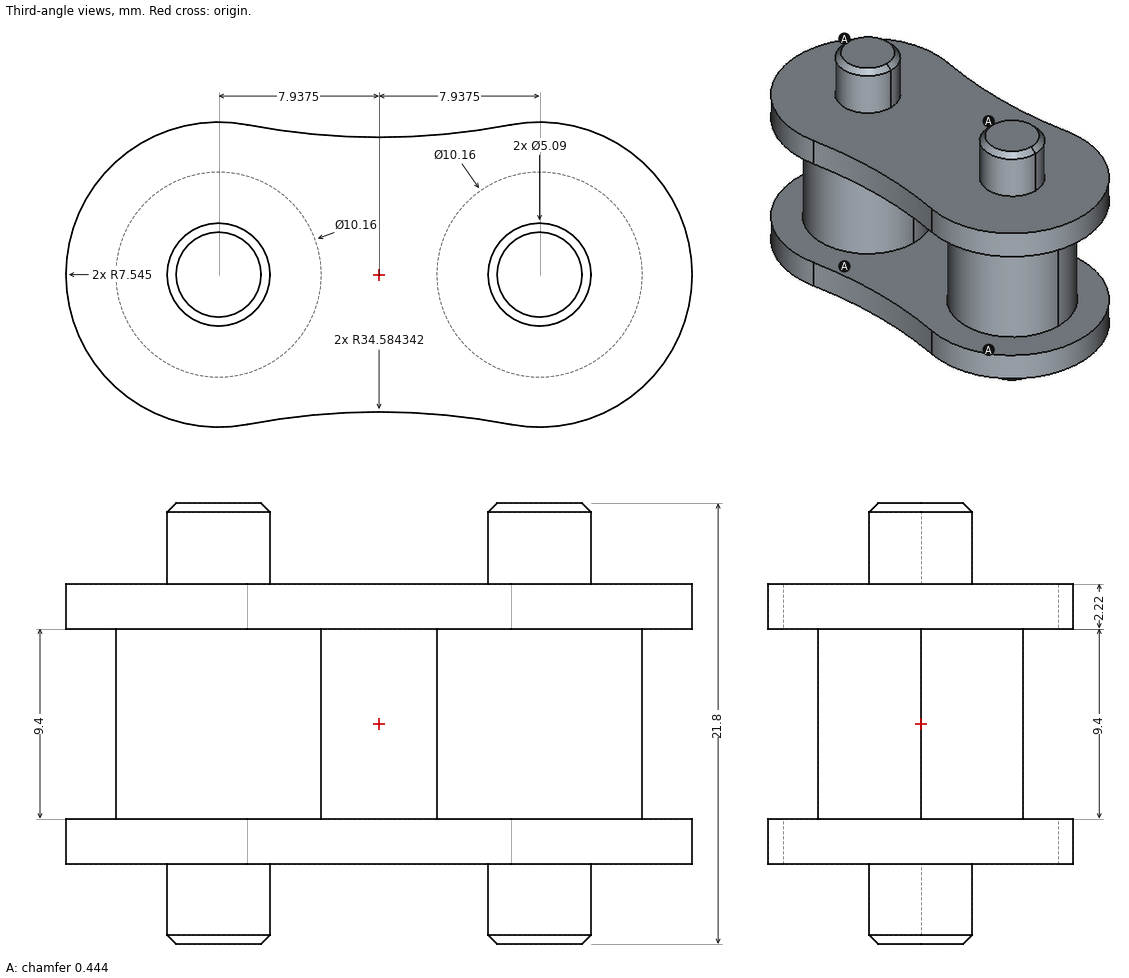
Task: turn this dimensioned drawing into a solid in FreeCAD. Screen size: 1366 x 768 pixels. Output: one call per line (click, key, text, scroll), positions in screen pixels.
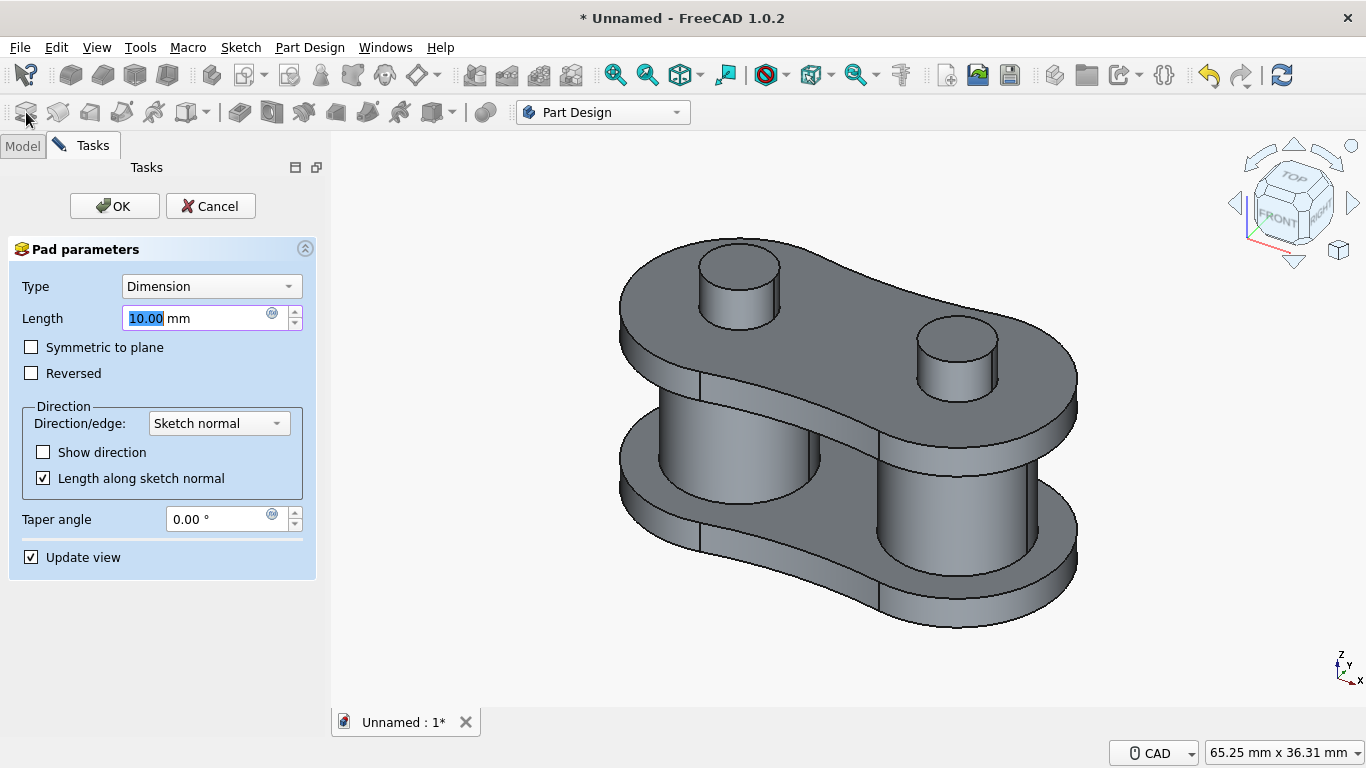
text(21.8)
key(Tab)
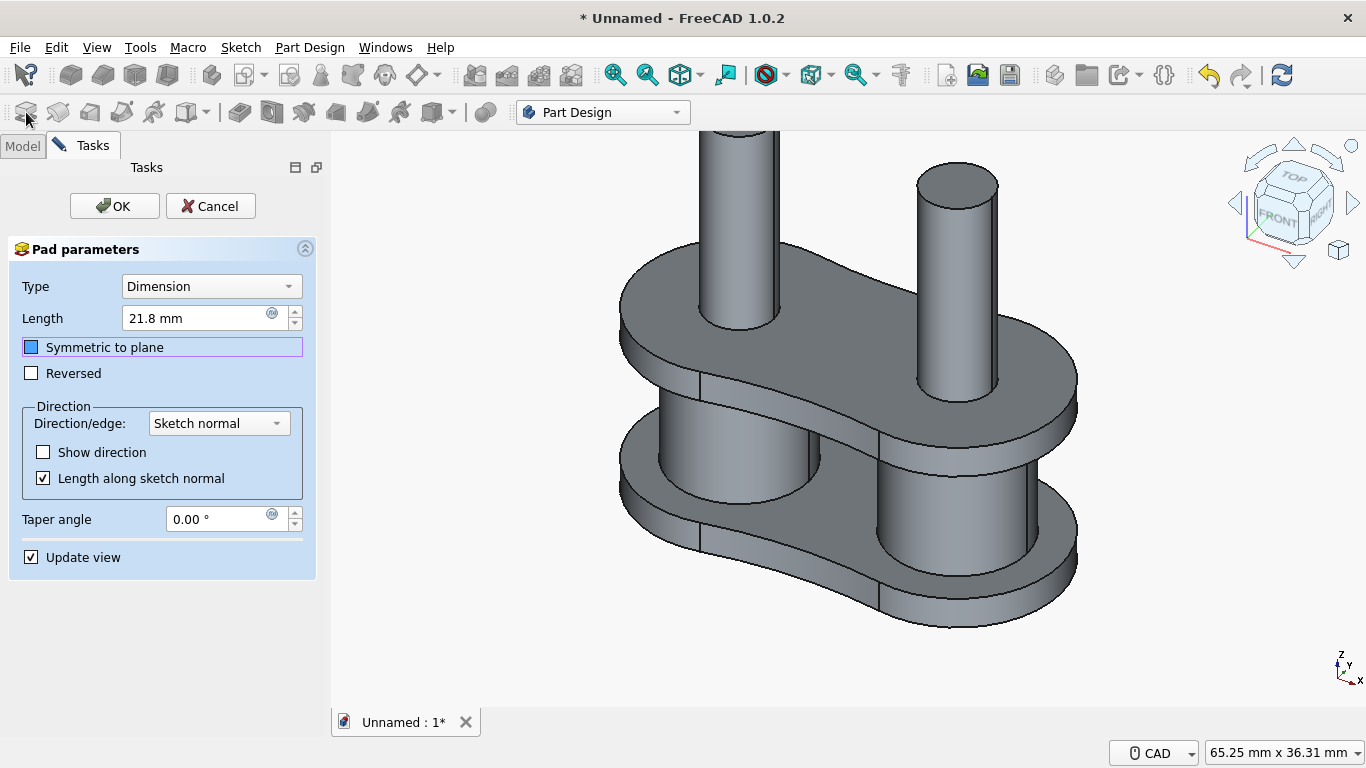
click(30, 347)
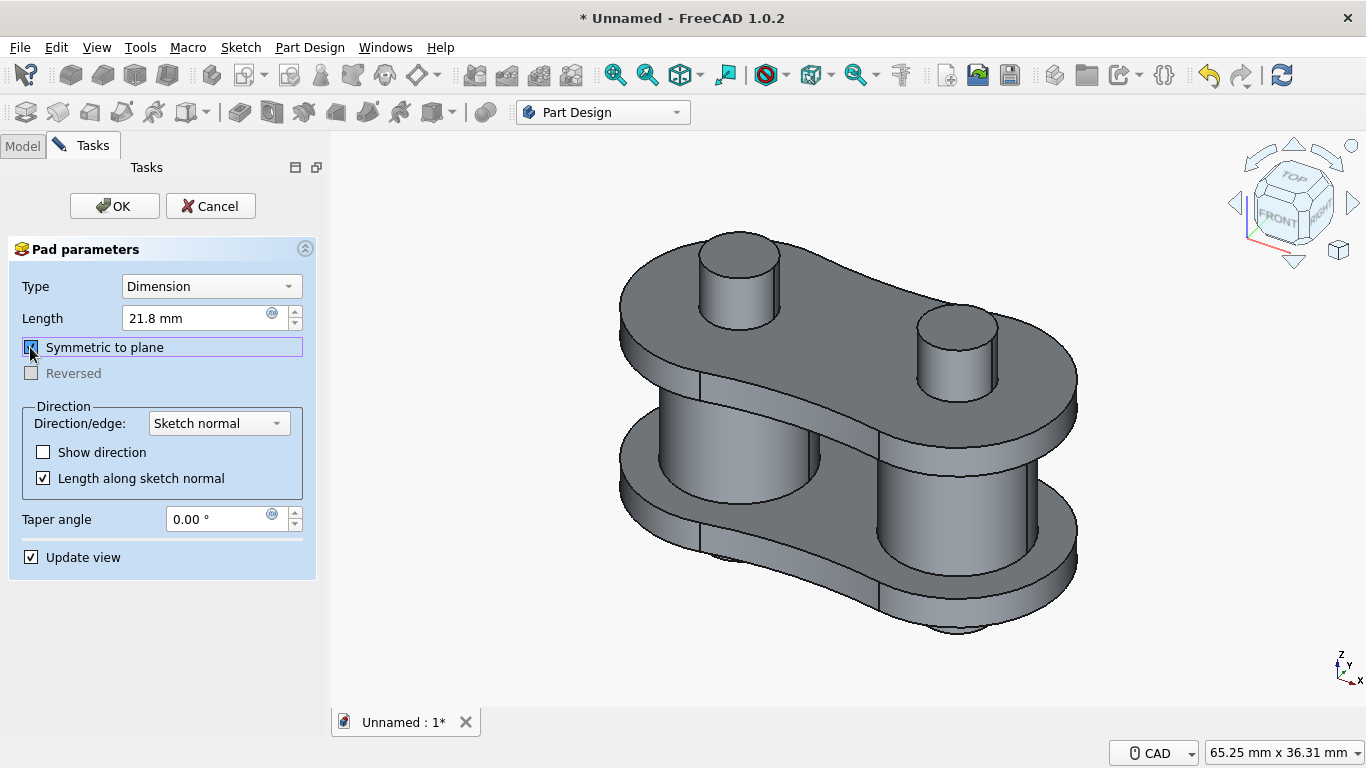
click(115, 206)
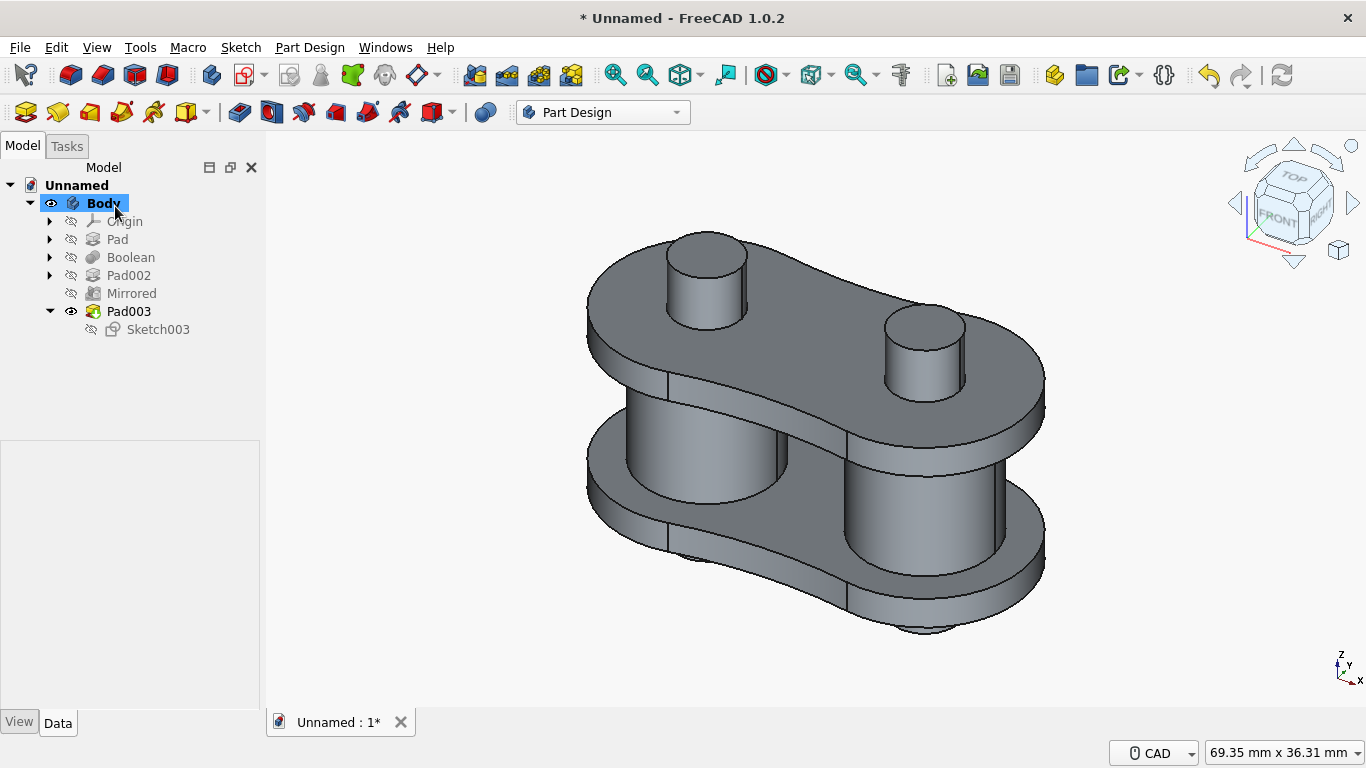
click(885, 329)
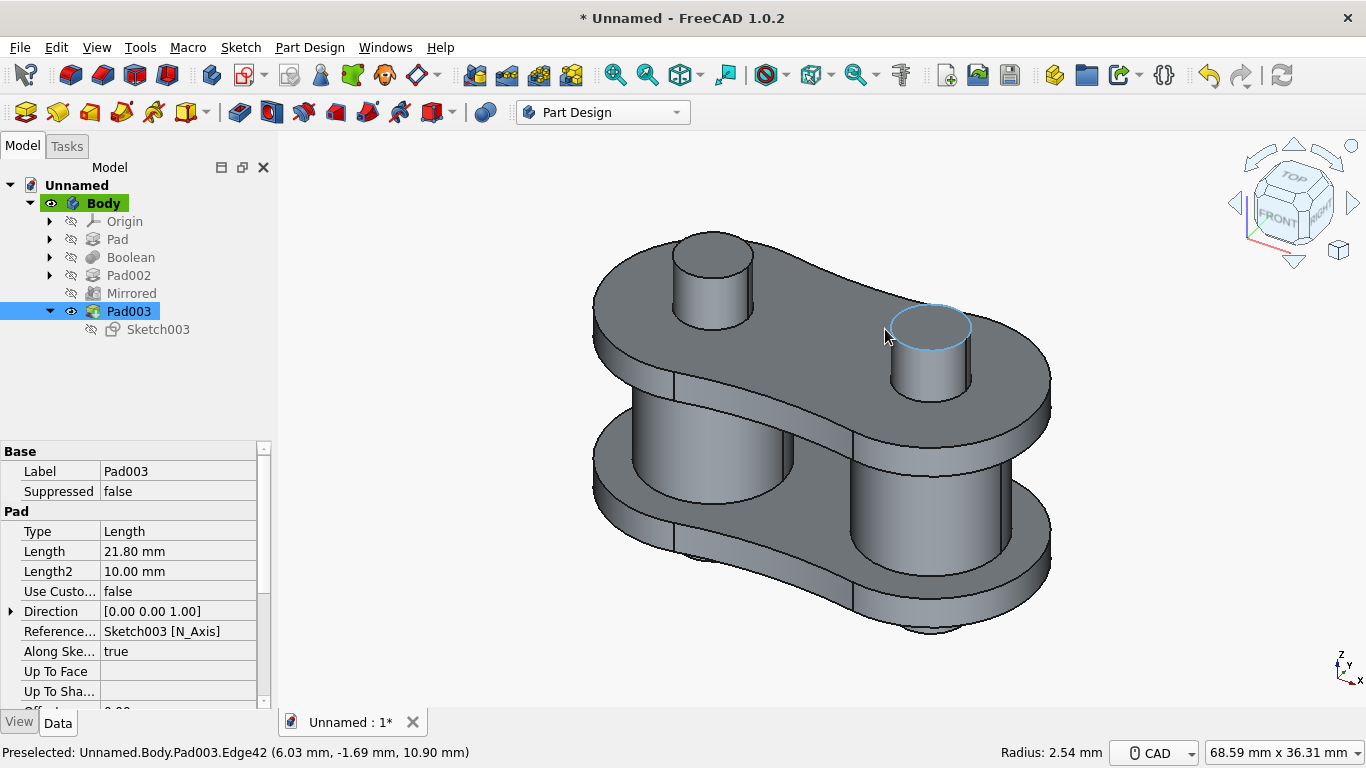
click(673, 257, ctrl)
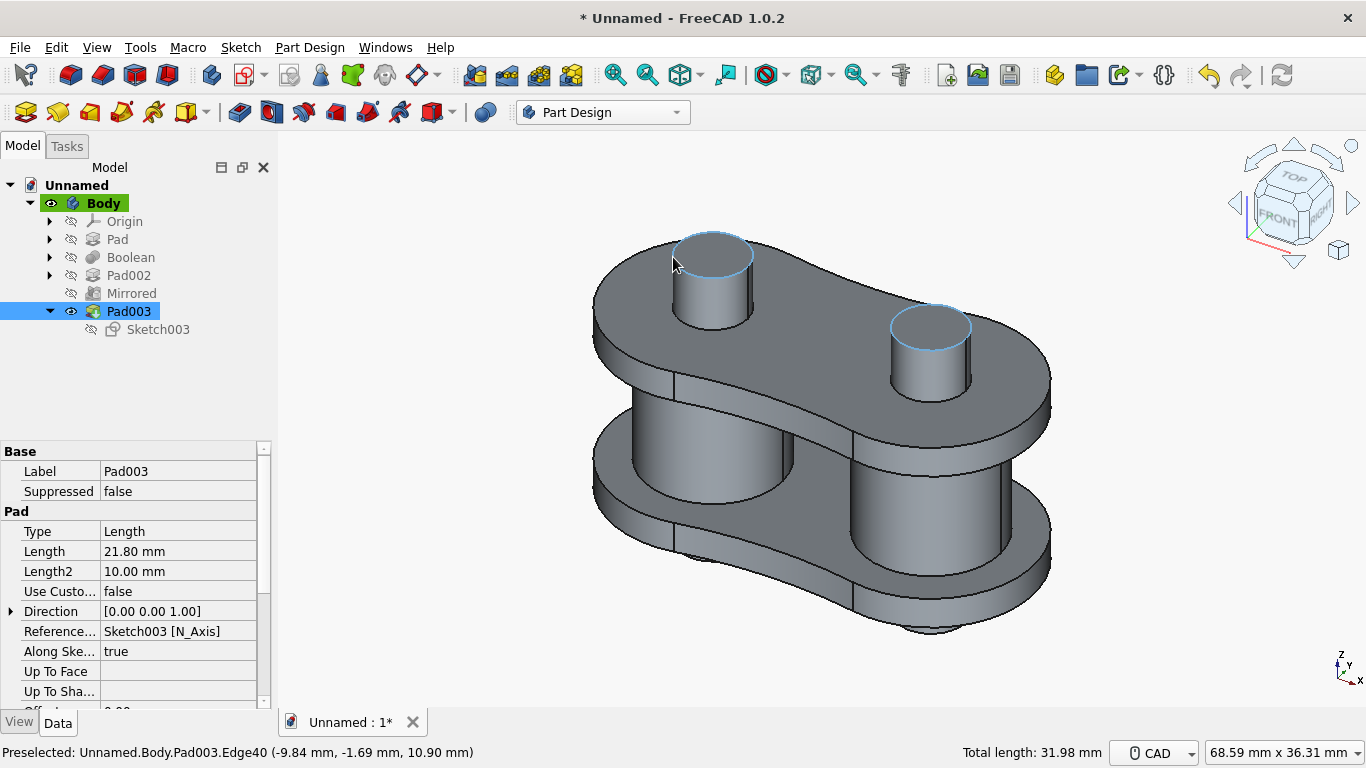
key(0)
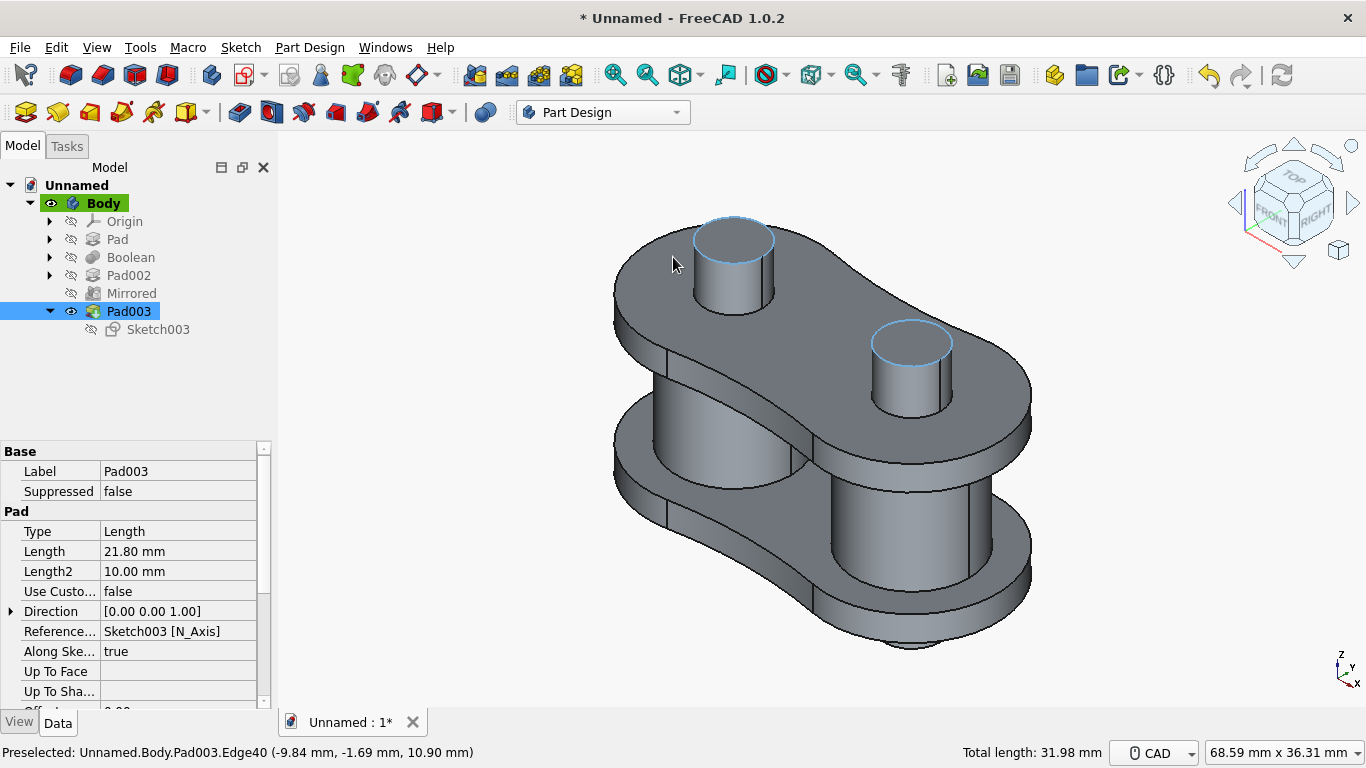
key(v)
key(f)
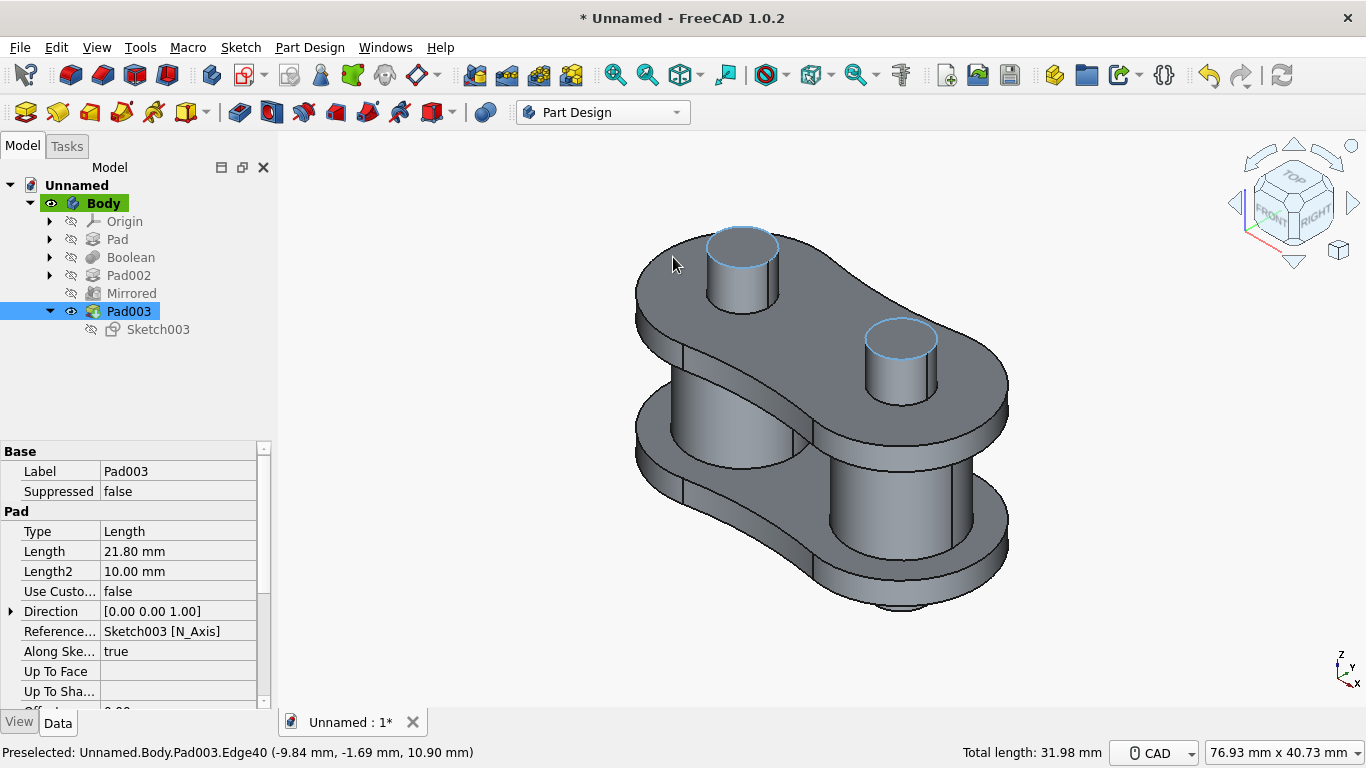
key(2)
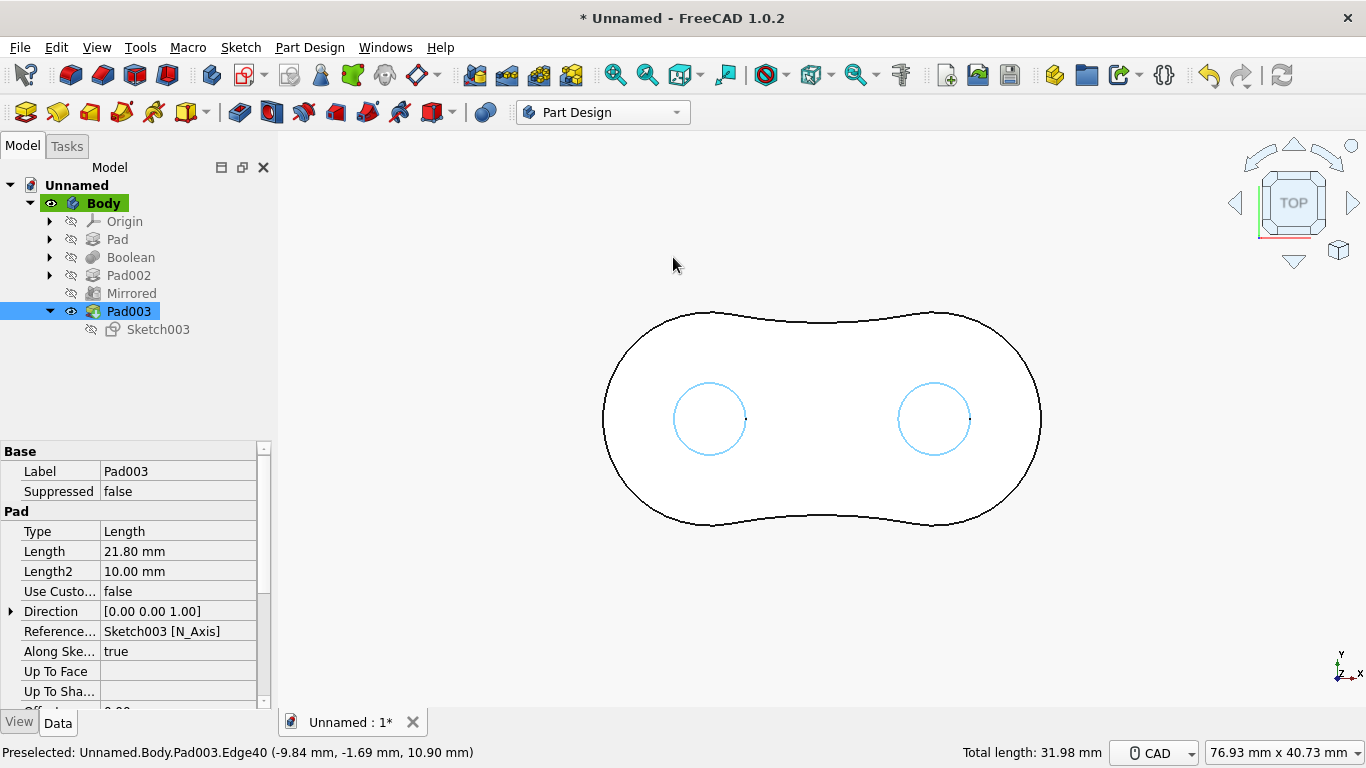
click(616, 76)